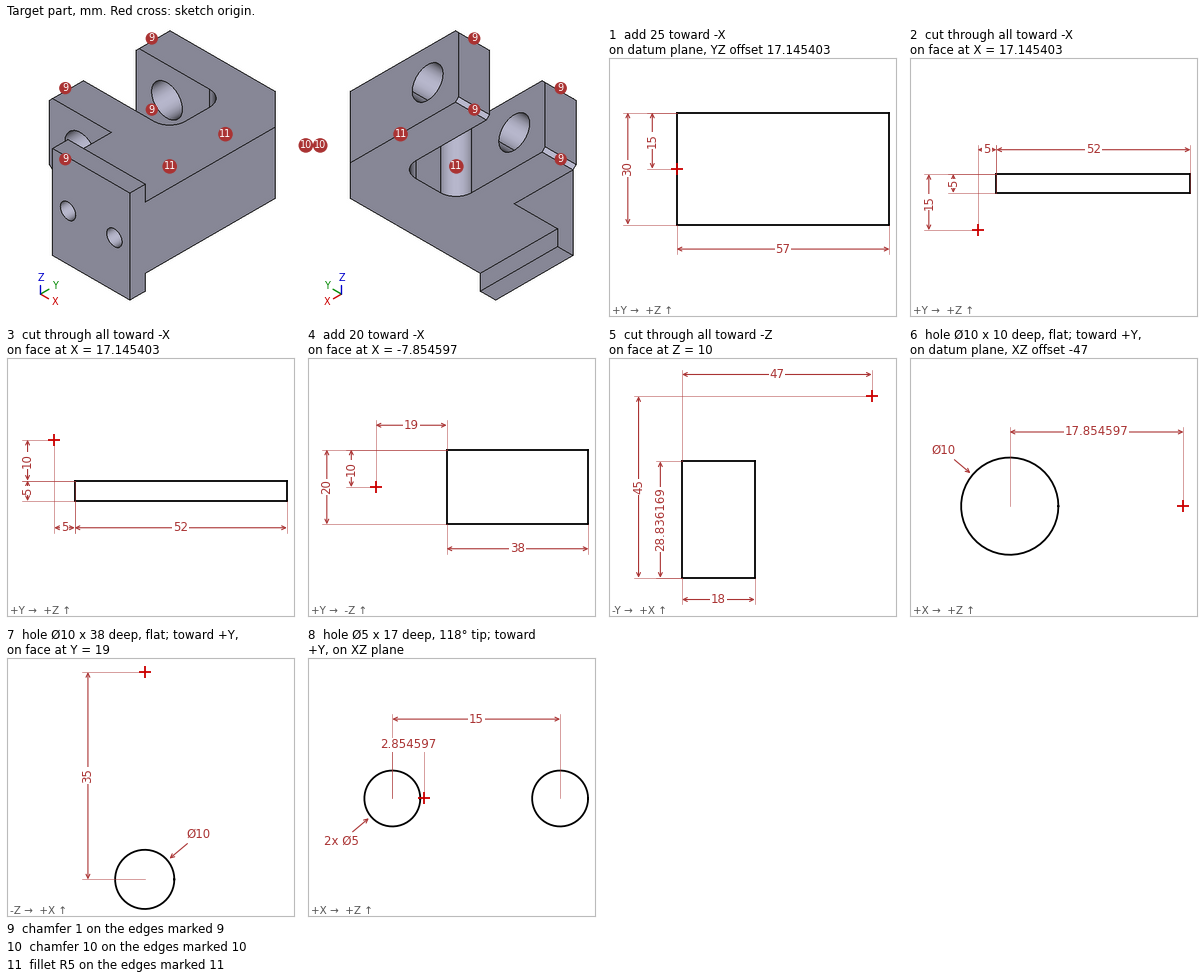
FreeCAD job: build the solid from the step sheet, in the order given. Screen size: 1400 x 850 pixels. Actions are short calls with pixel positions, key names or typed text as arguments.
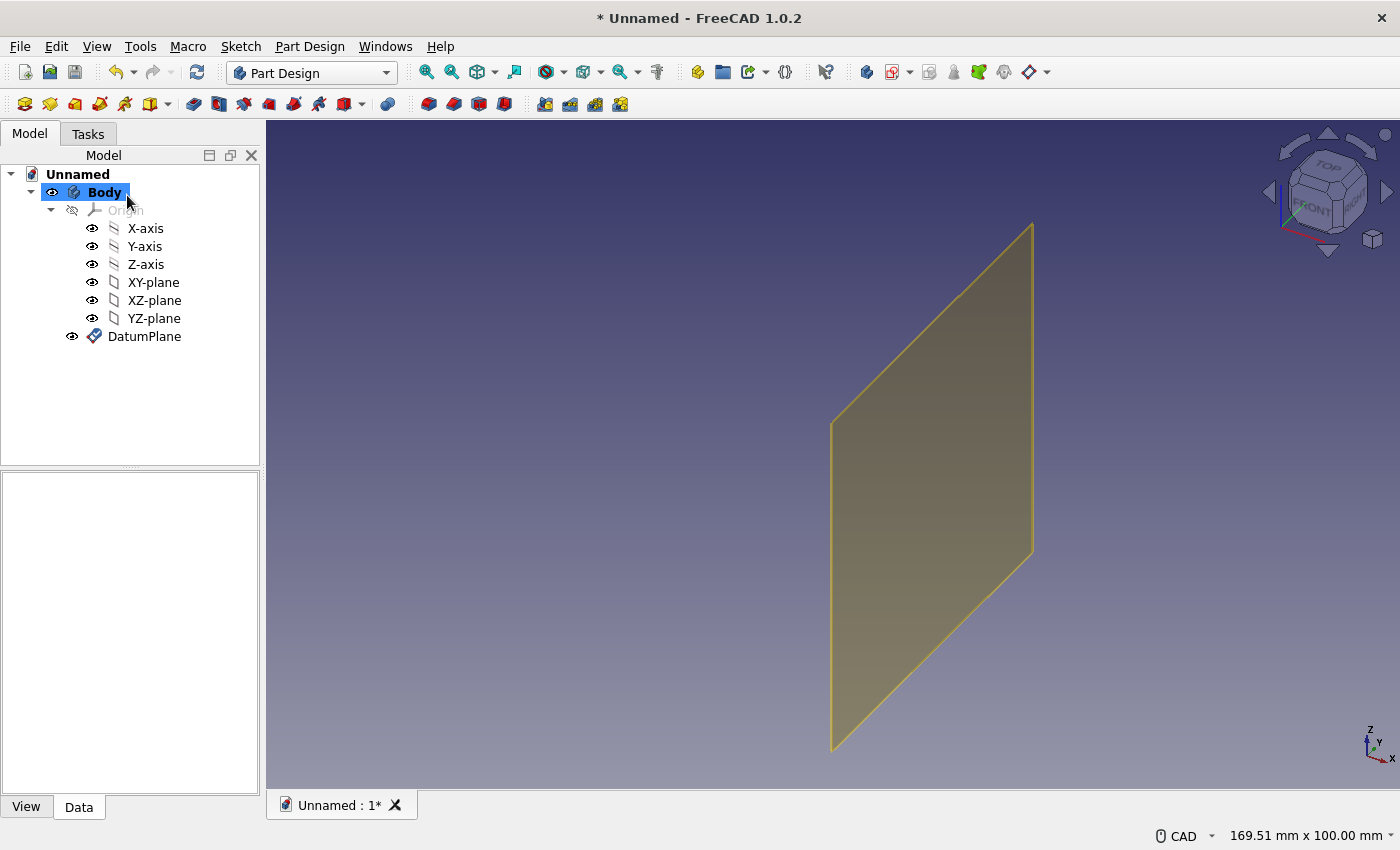
click(117, 336)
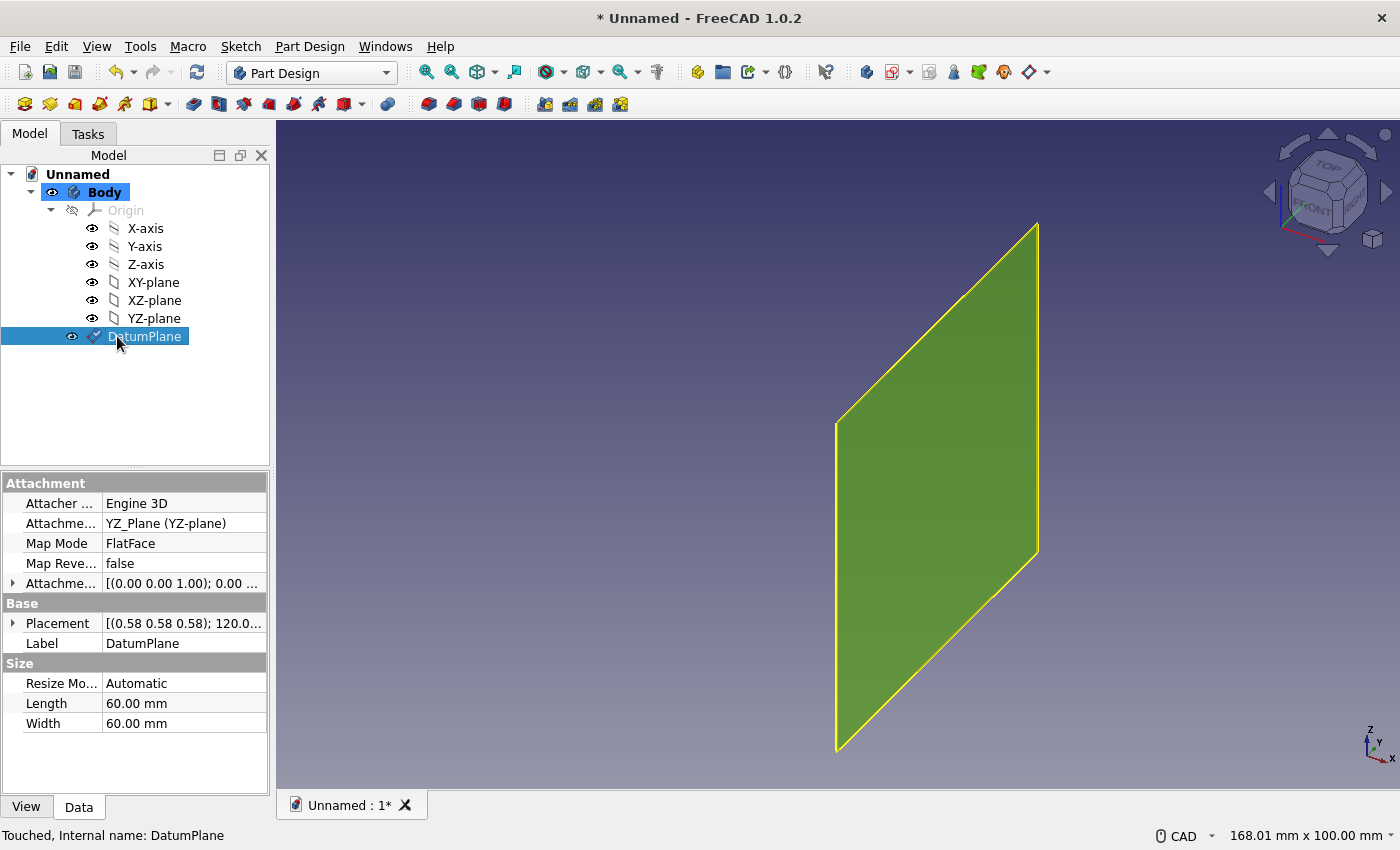
click(892, 72)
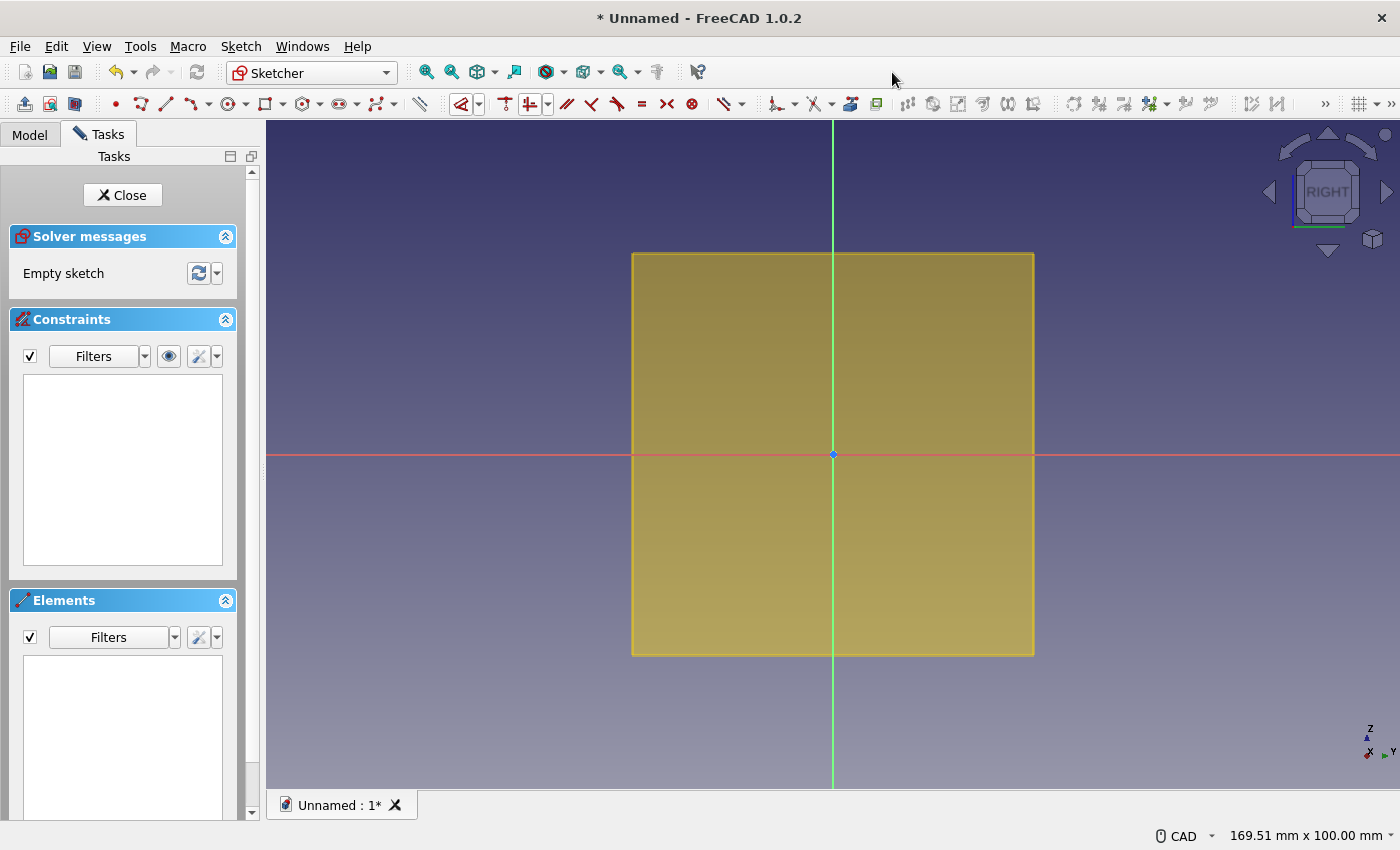
scroll(1235, 454, up, 3)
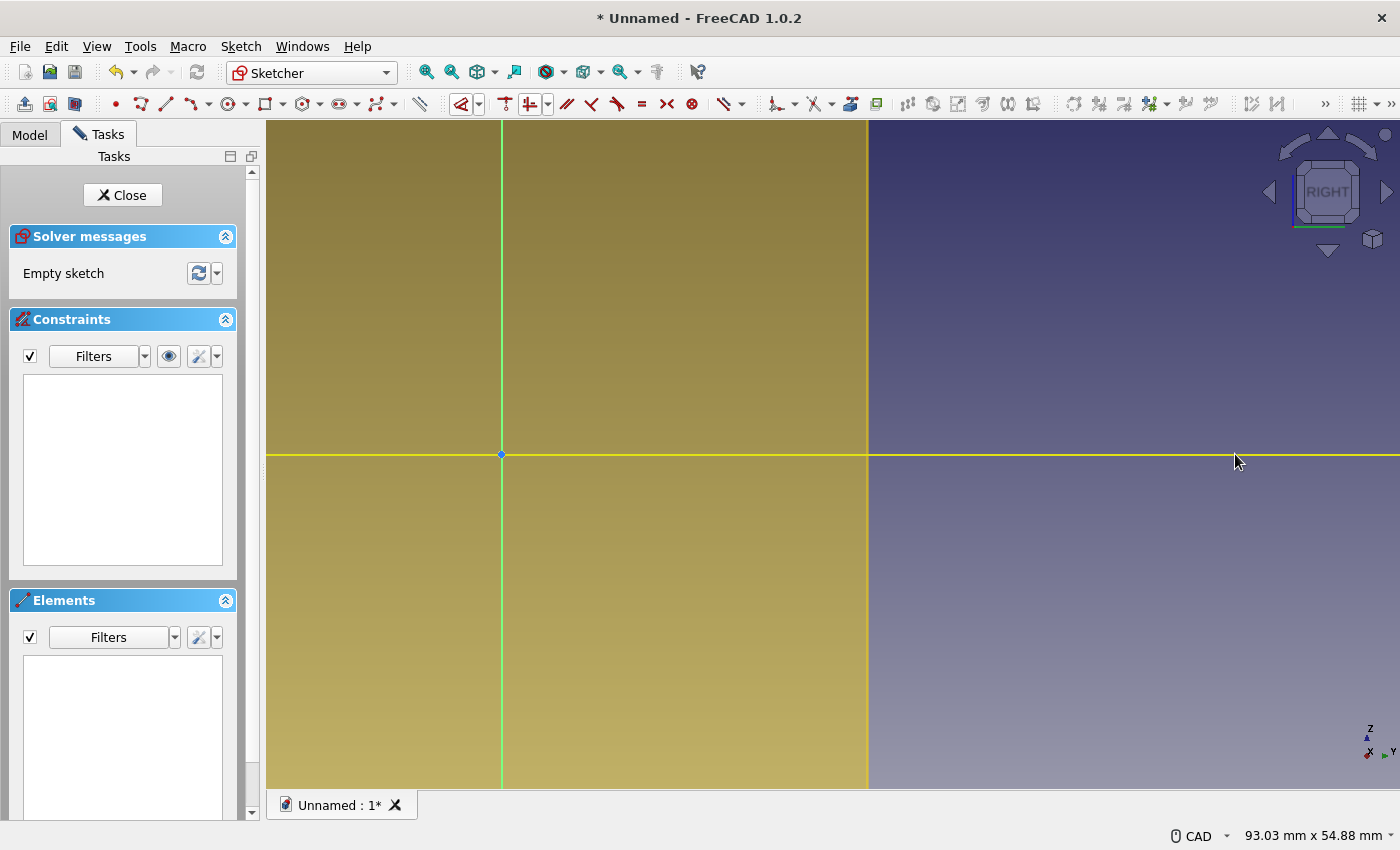
click(264, 104)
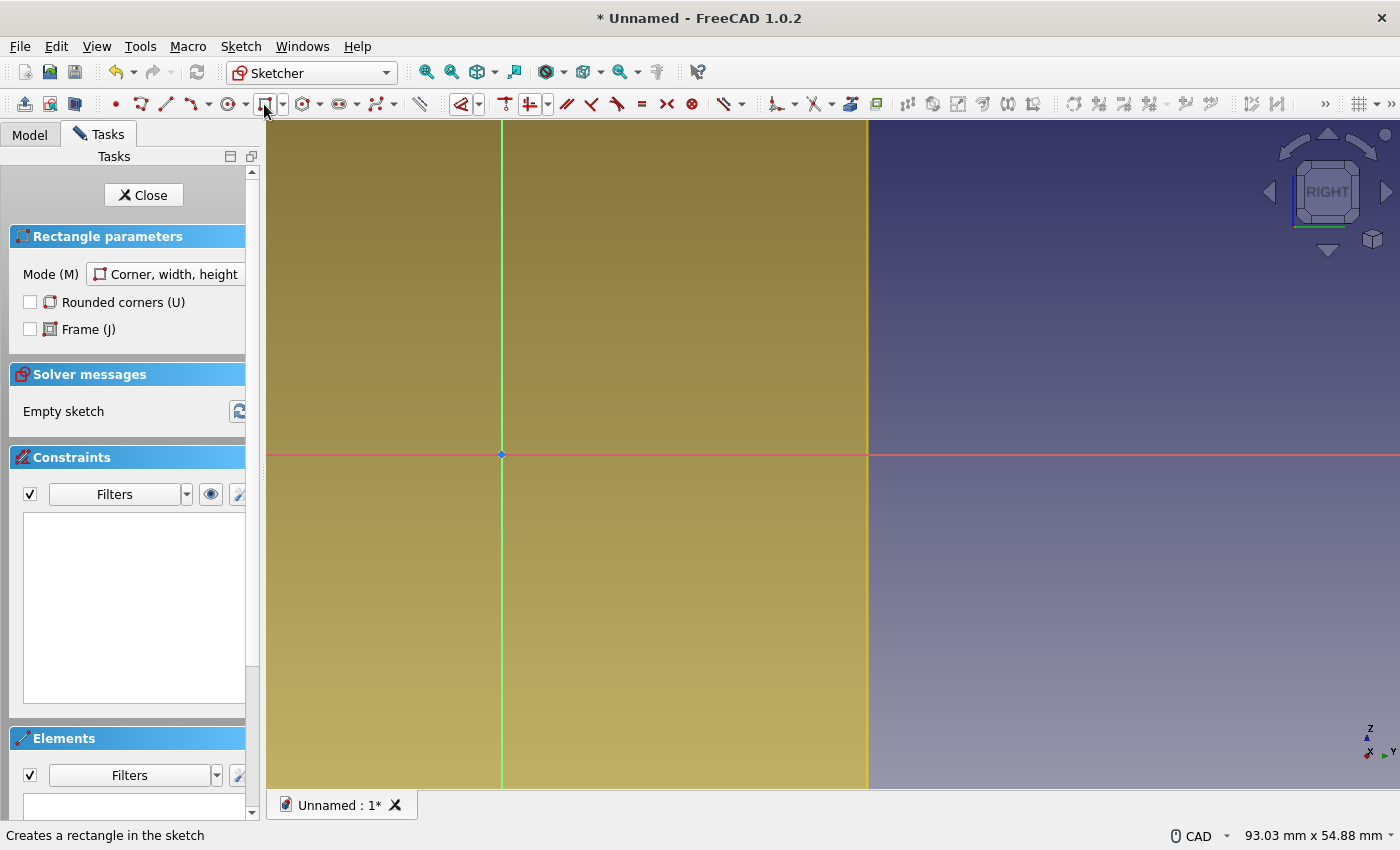
click(502, 272)
click(1197, 637)
key(Escape)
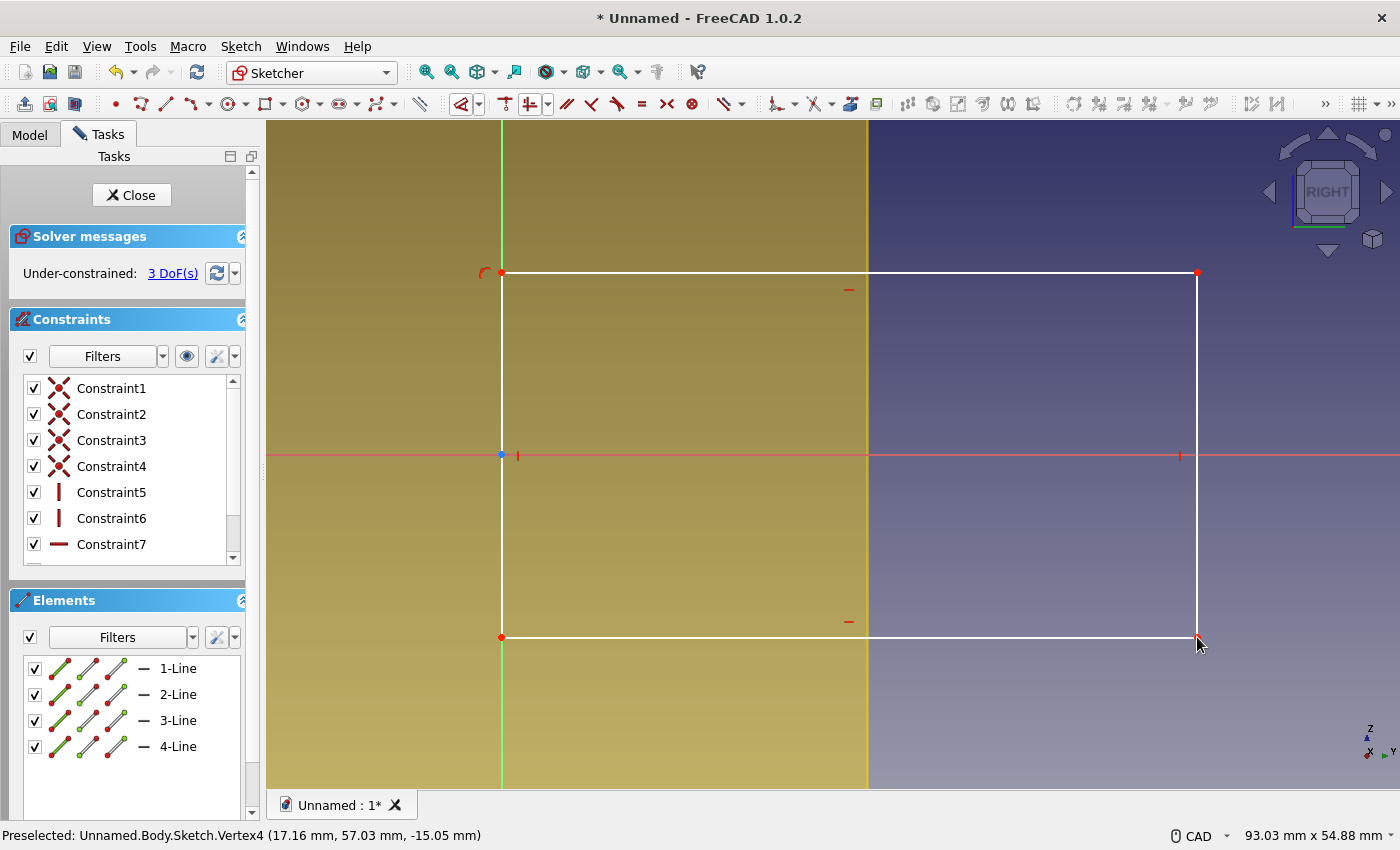
key(d)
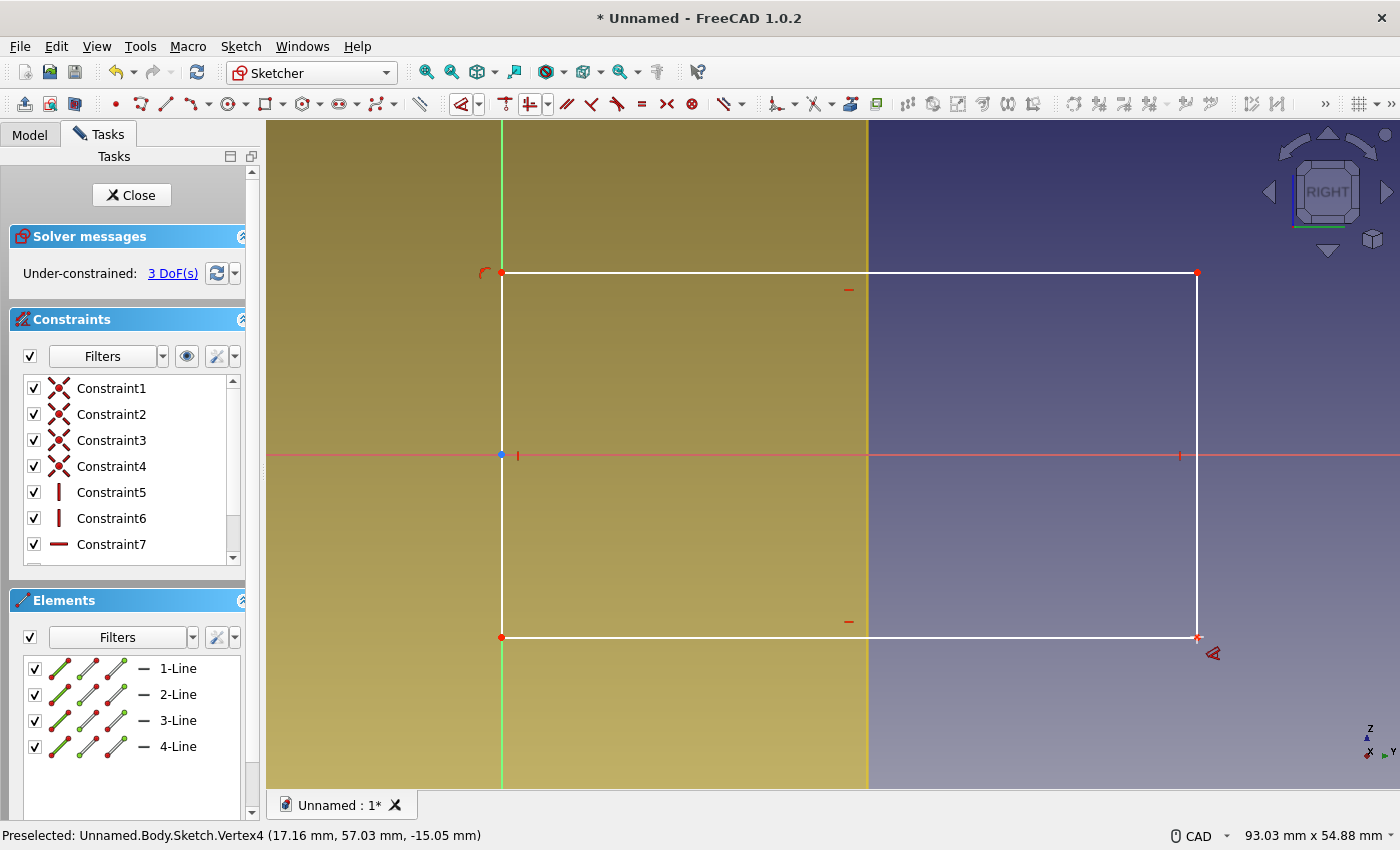
click(502, 383)
click(468, 372)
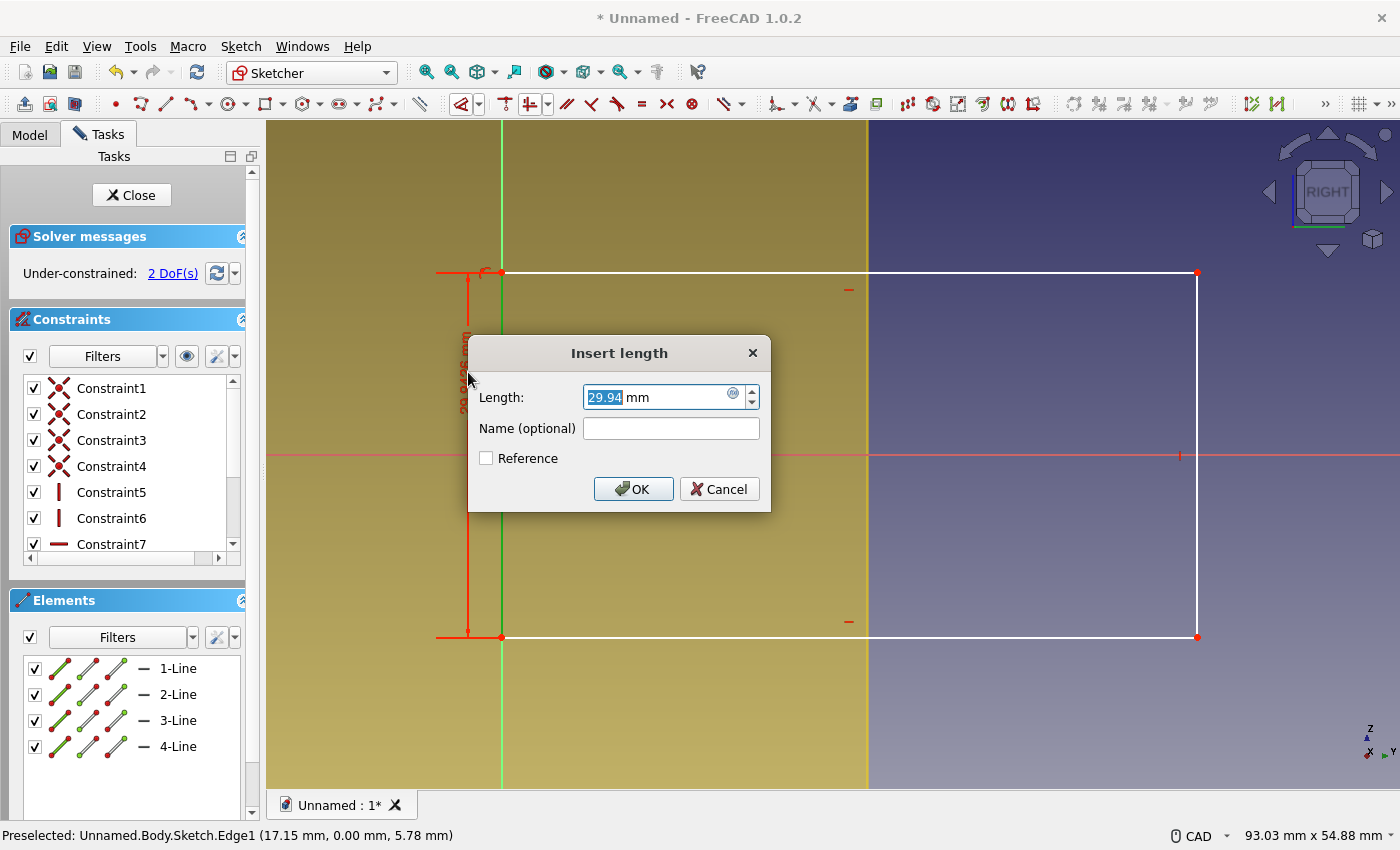
text(30)
key(Return)